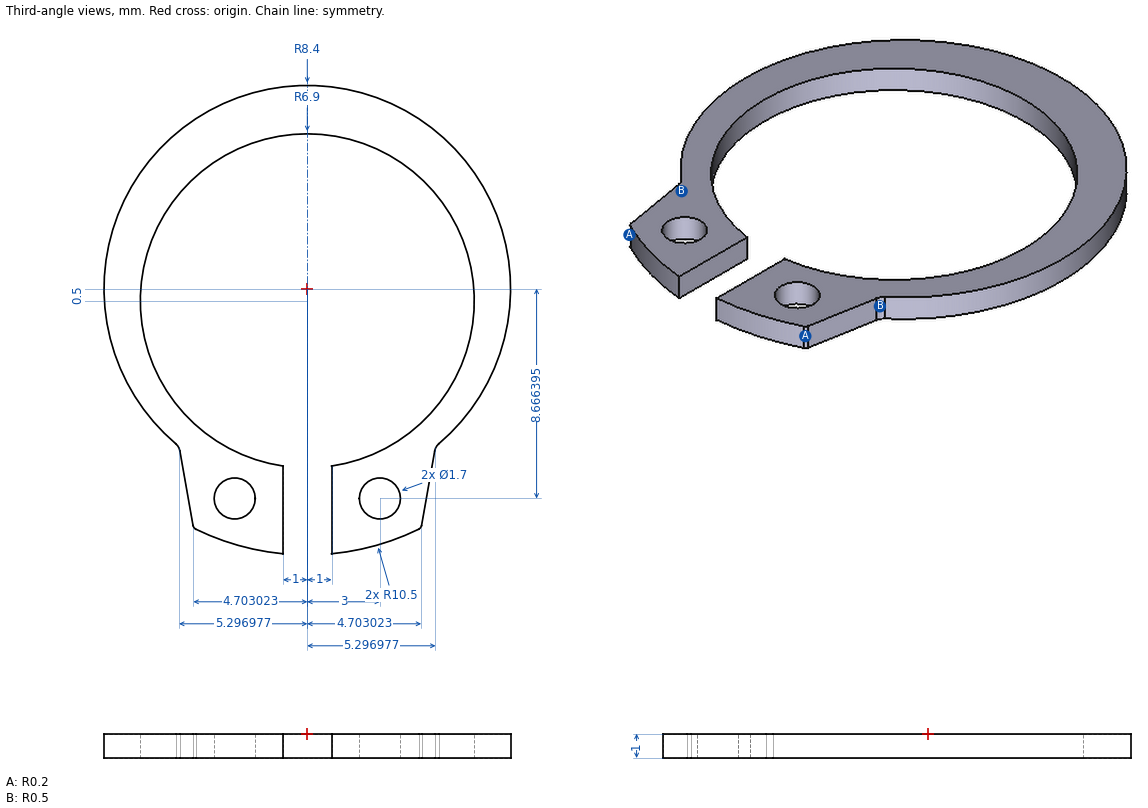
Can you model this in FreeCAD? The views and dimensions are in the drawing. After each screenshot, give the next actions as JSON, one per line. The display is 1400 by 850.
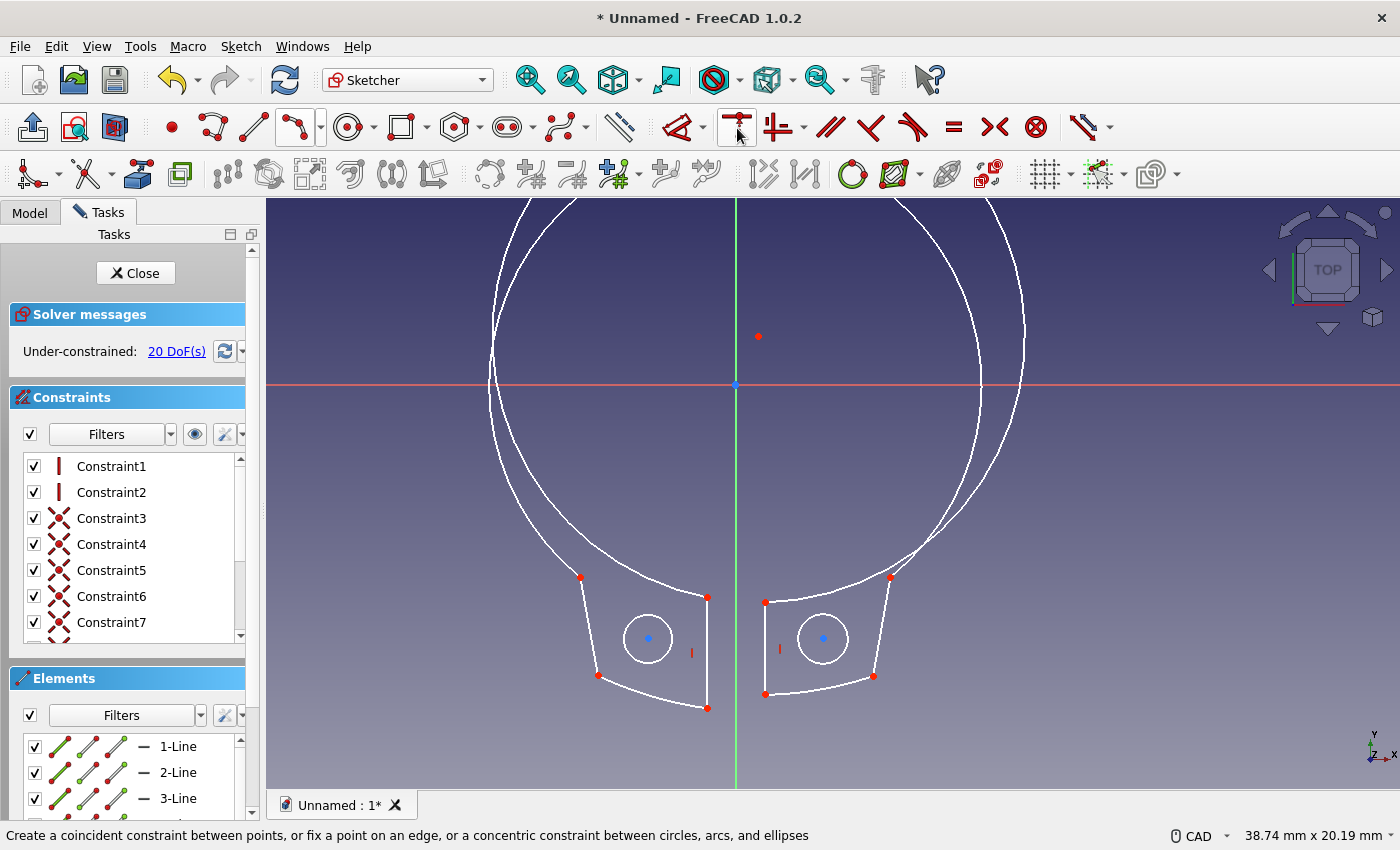
{"action": "scroll", "coordinate": [735, 385], "scroll_direction": "up", "scroll_amount": 3}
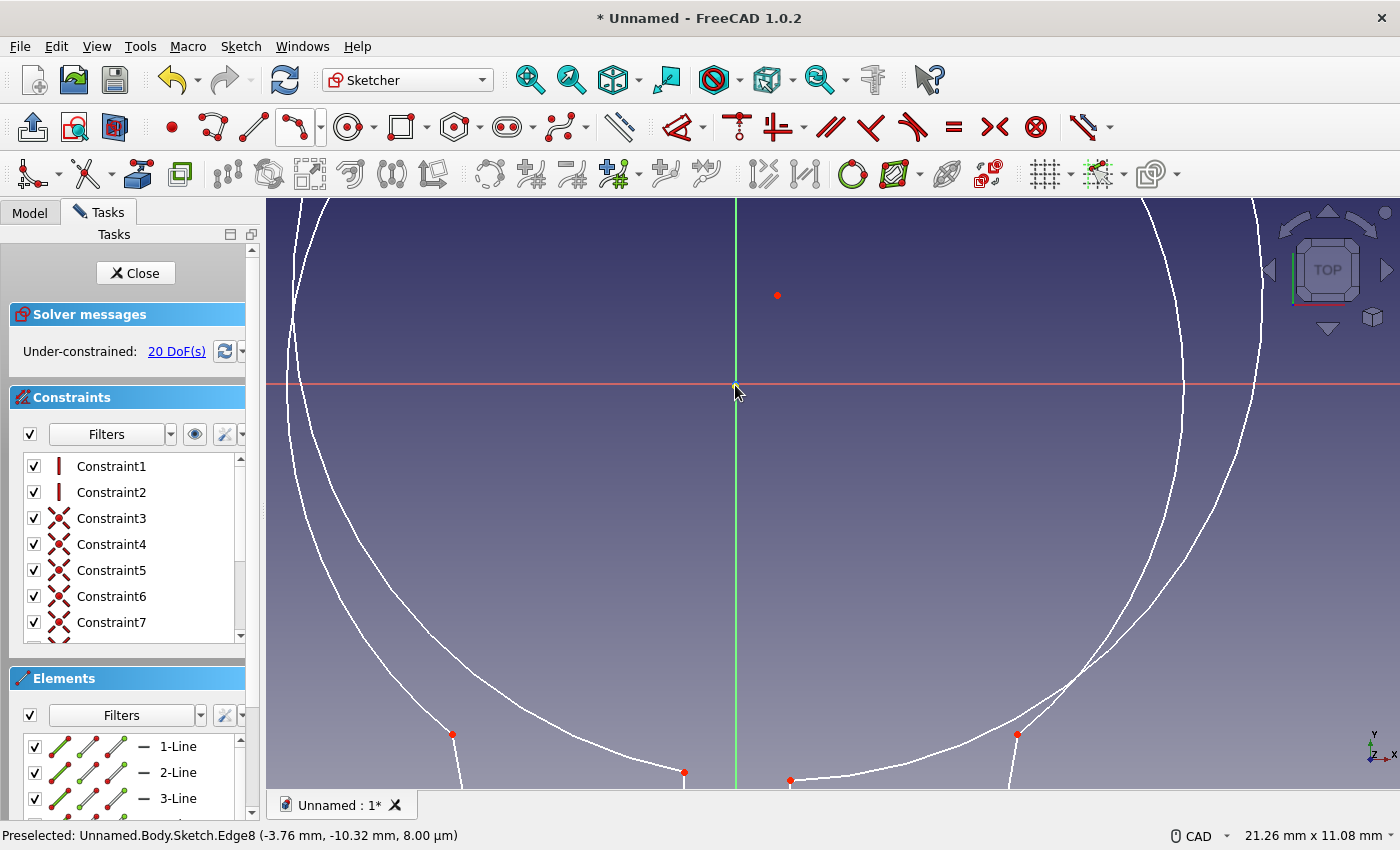
{"action": "left_click_drag", "start_coordinate": [725, 374], "coordinate": [746, 397]}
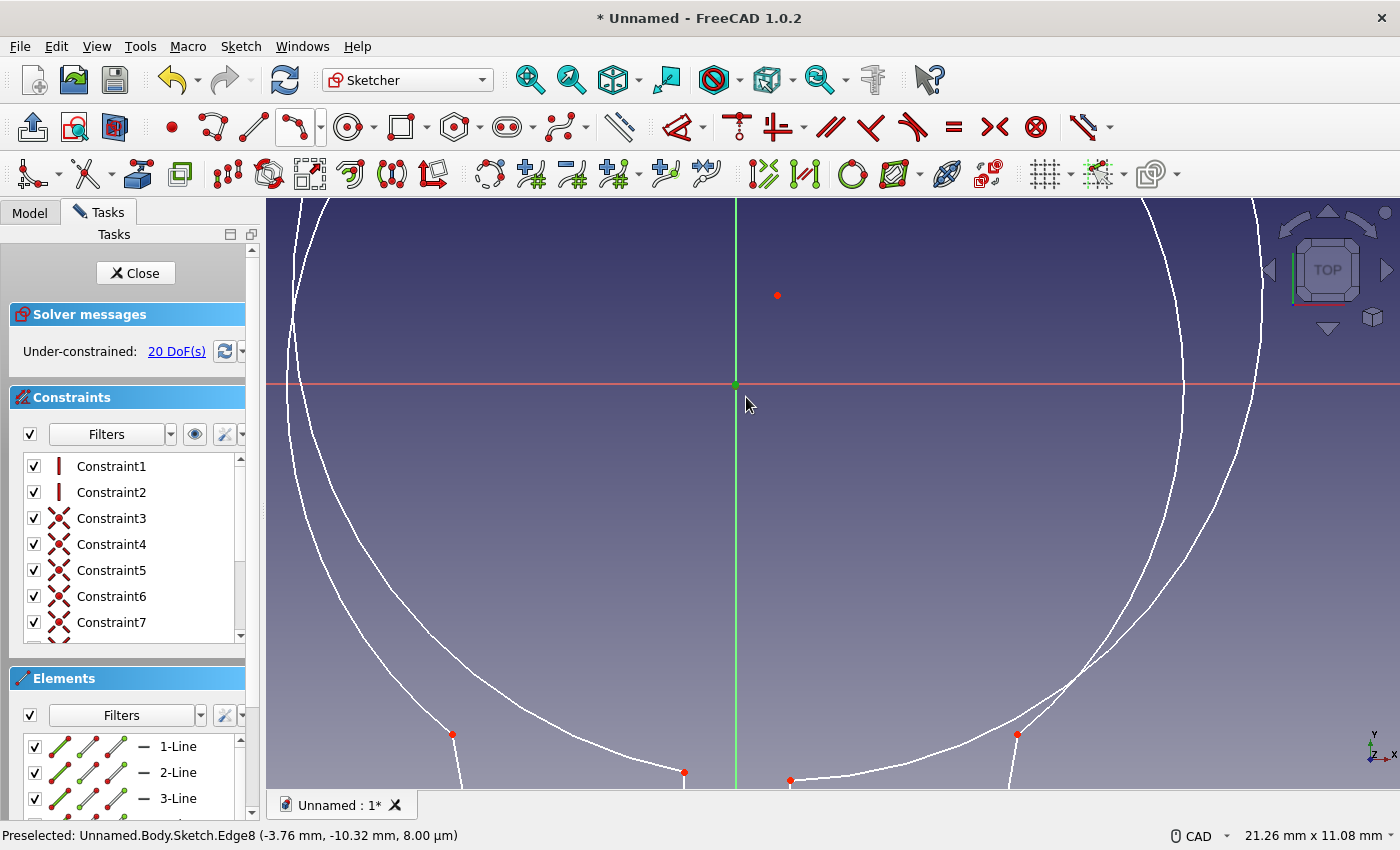
{"action": "left_click", "coordinate": [737, 128]}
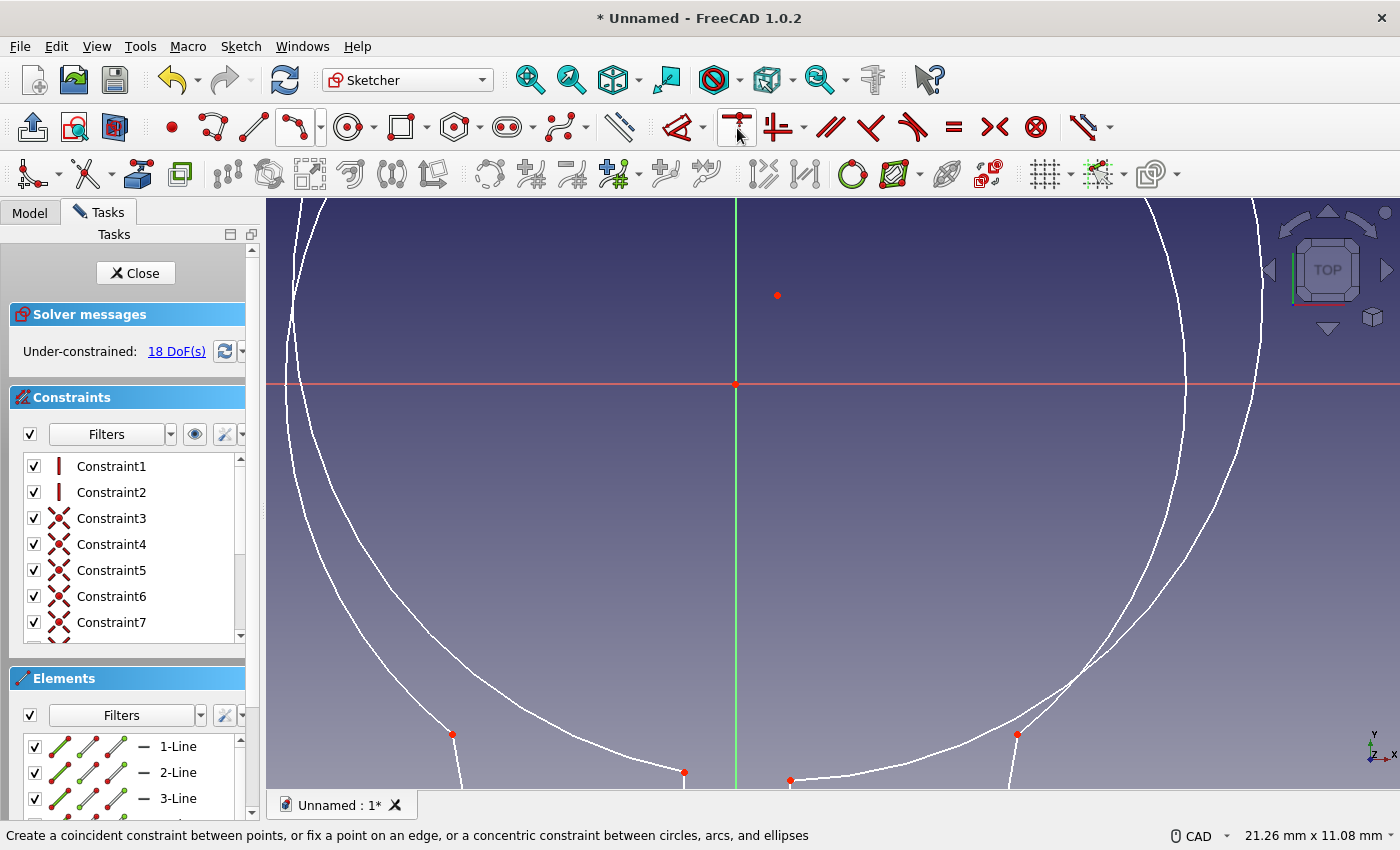
{"action": "scroll", "coordinate": [781, 518], "scroll_direction": "down", "scroll_amount": 5}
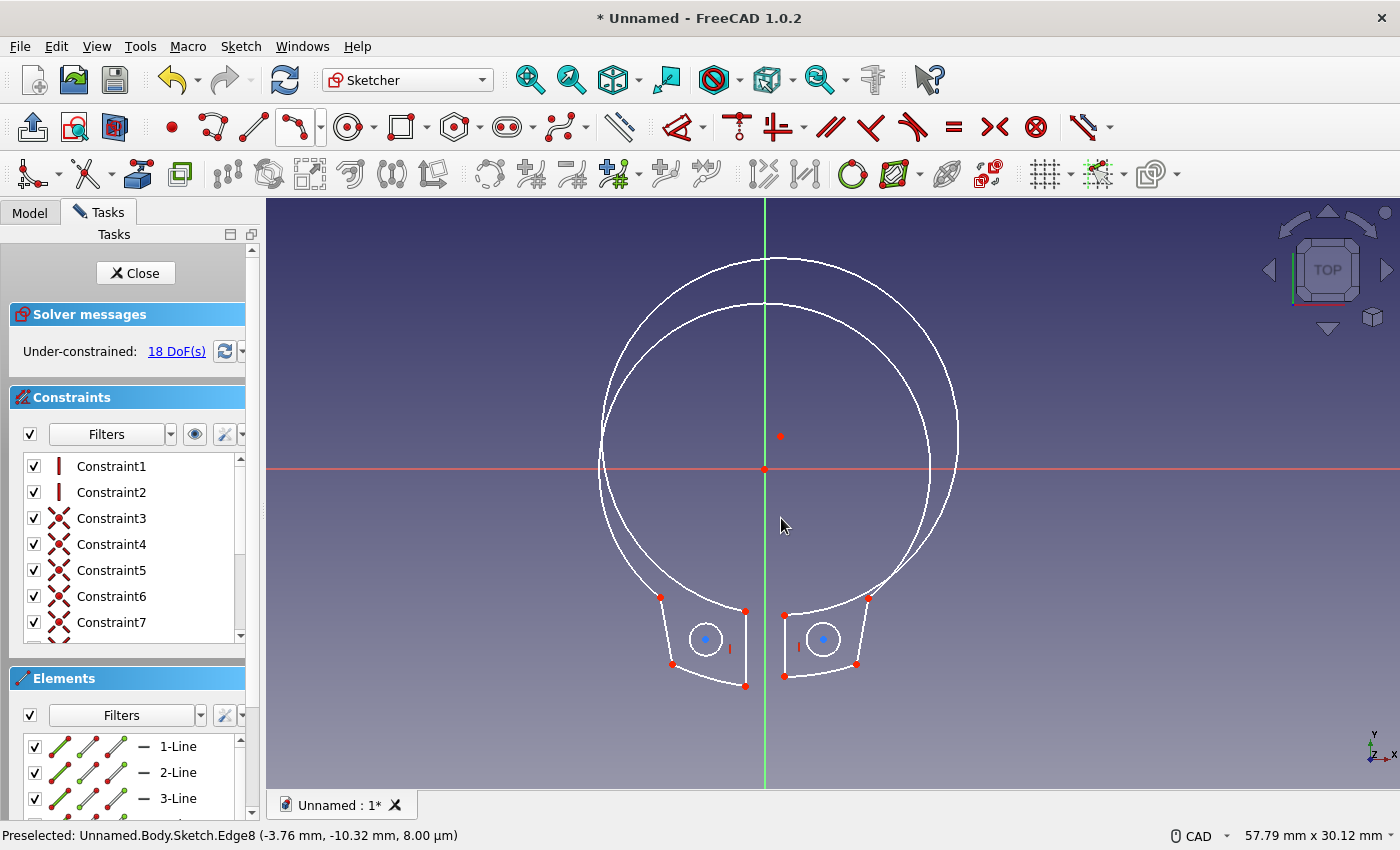
{"action": "left_click", "coordinate": [807, 676]}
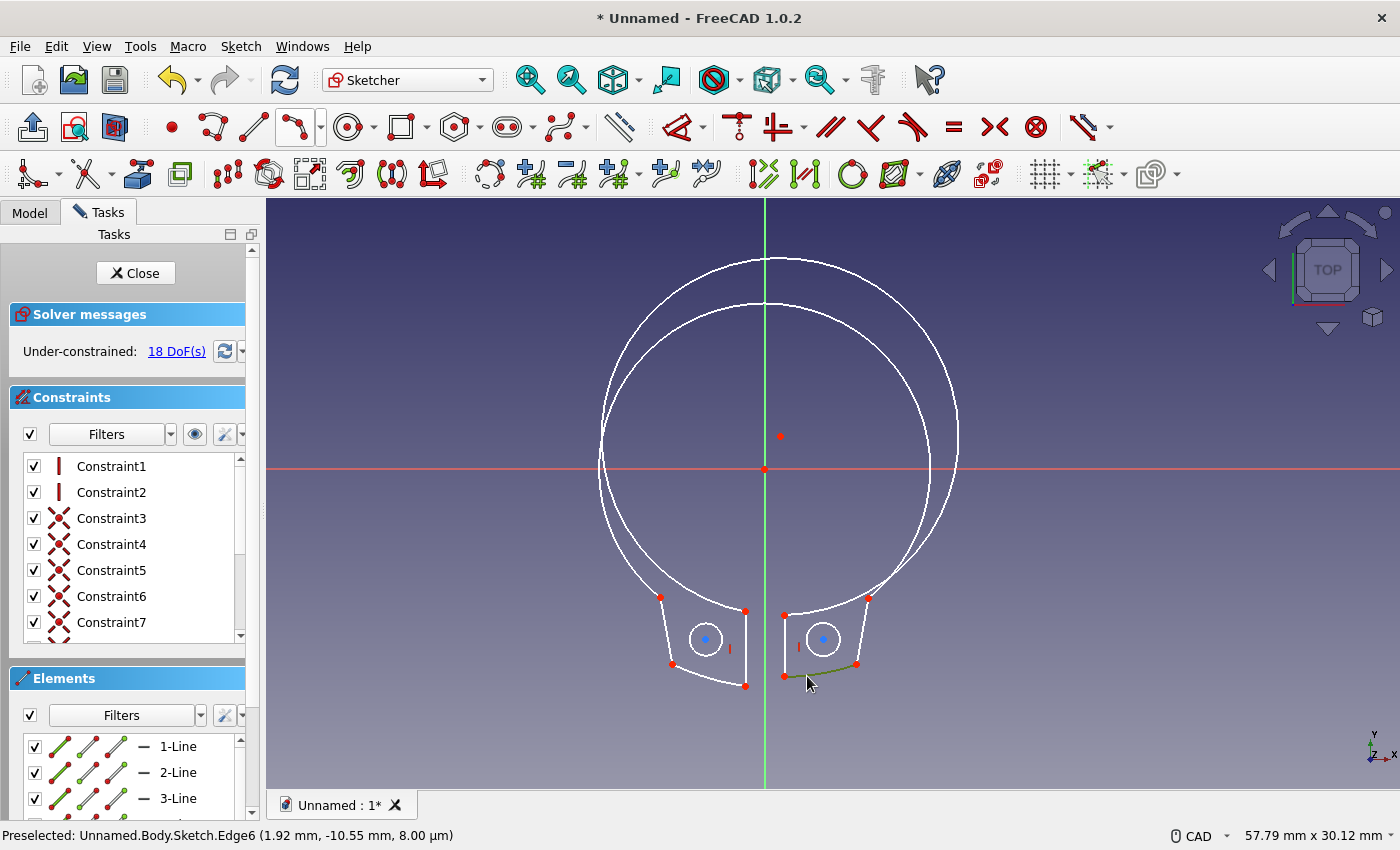
{"action": "left_click", "coordinate": [694, 673]}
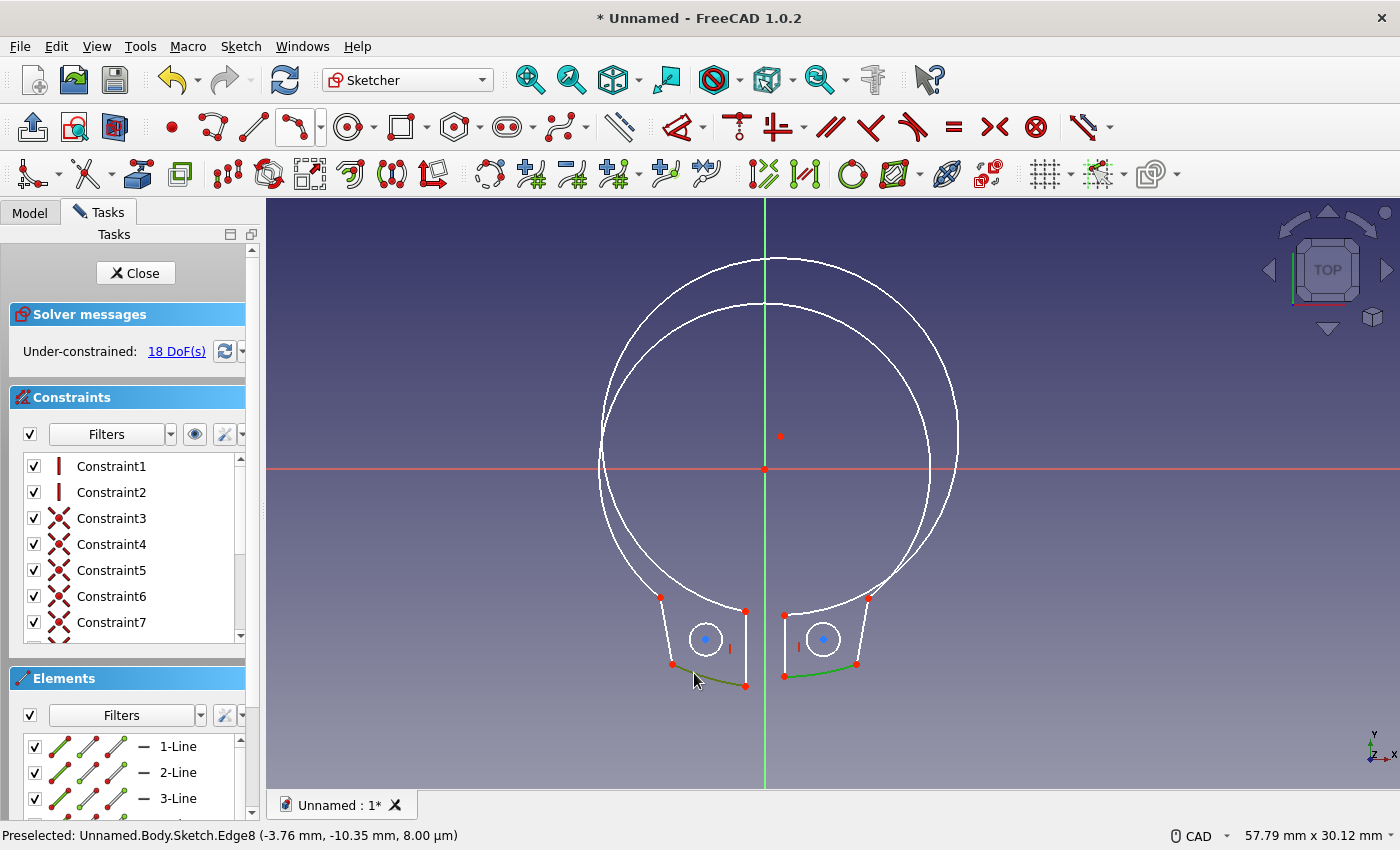
{"action": "left_click", "coordinate": [954, 128]}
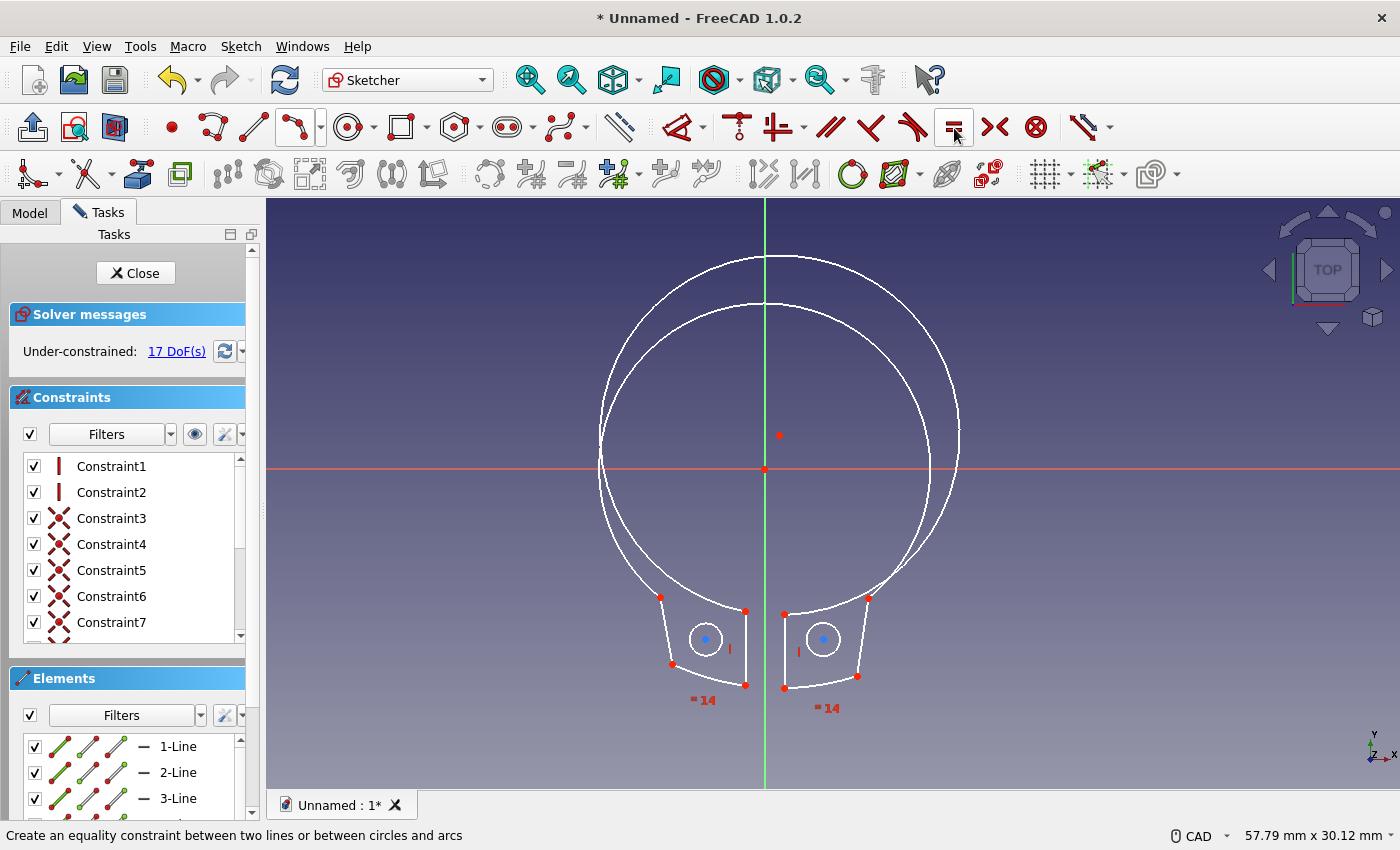
{"action": "left_click", "coordinate": [835, 628]}